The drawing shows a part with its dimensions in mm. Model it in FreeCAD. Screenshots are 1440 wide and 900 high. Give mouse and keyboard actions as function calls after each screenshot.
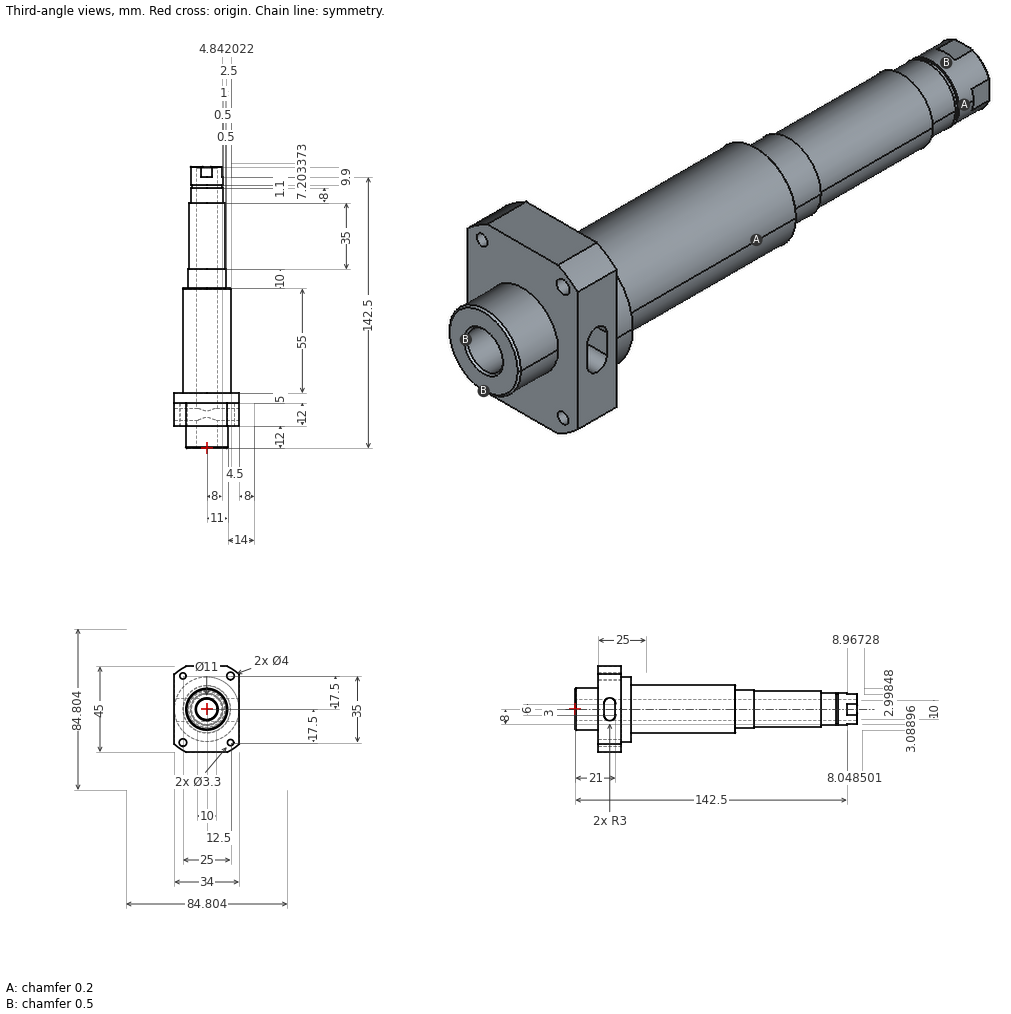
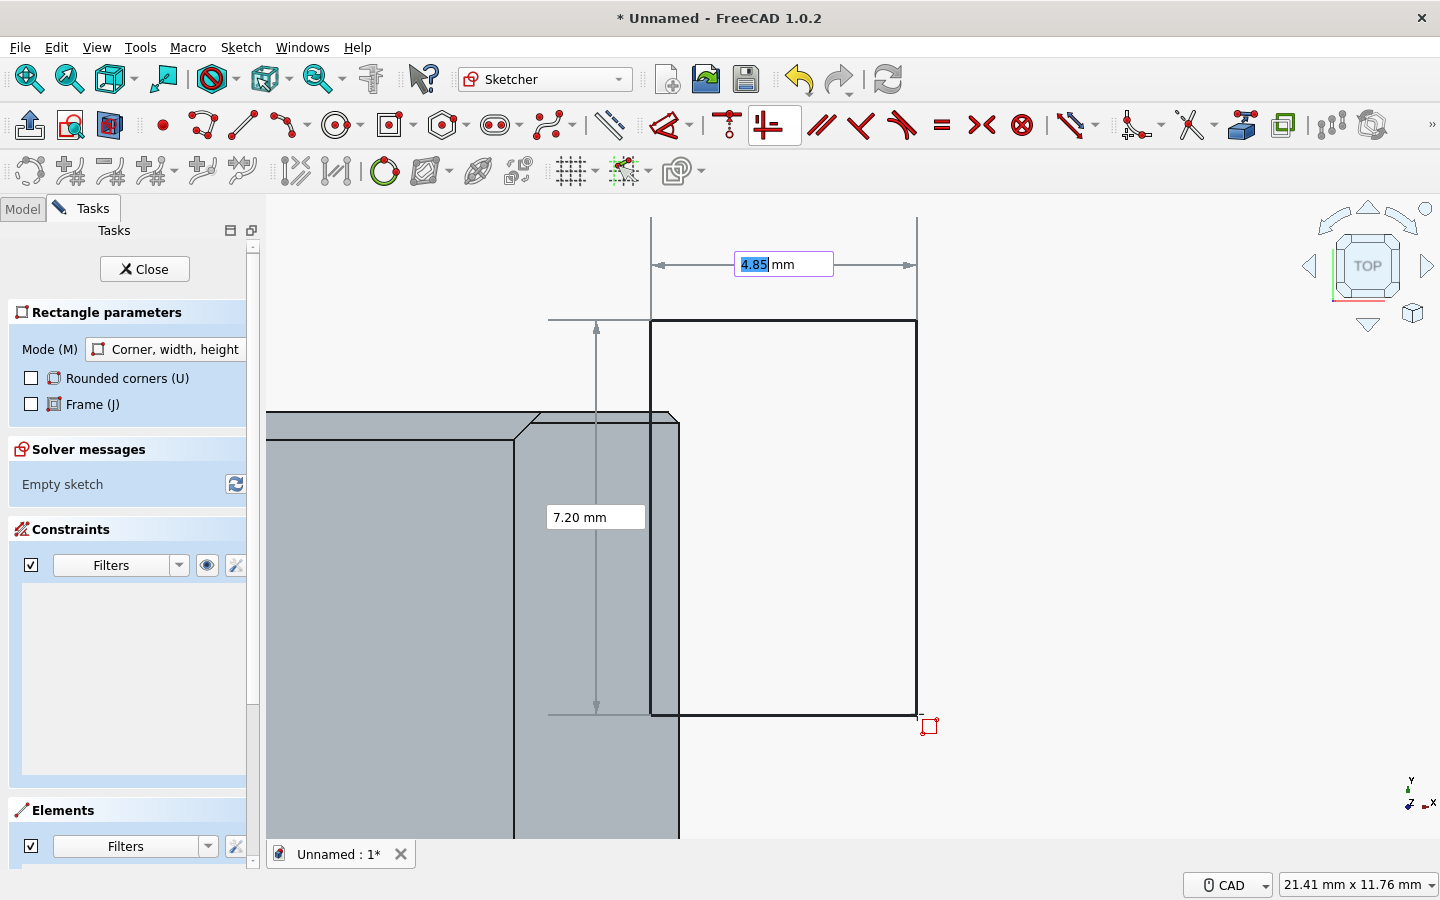
text(4.842022)
key(Tab)
text(7.203373)
key(Return)
key(Escape)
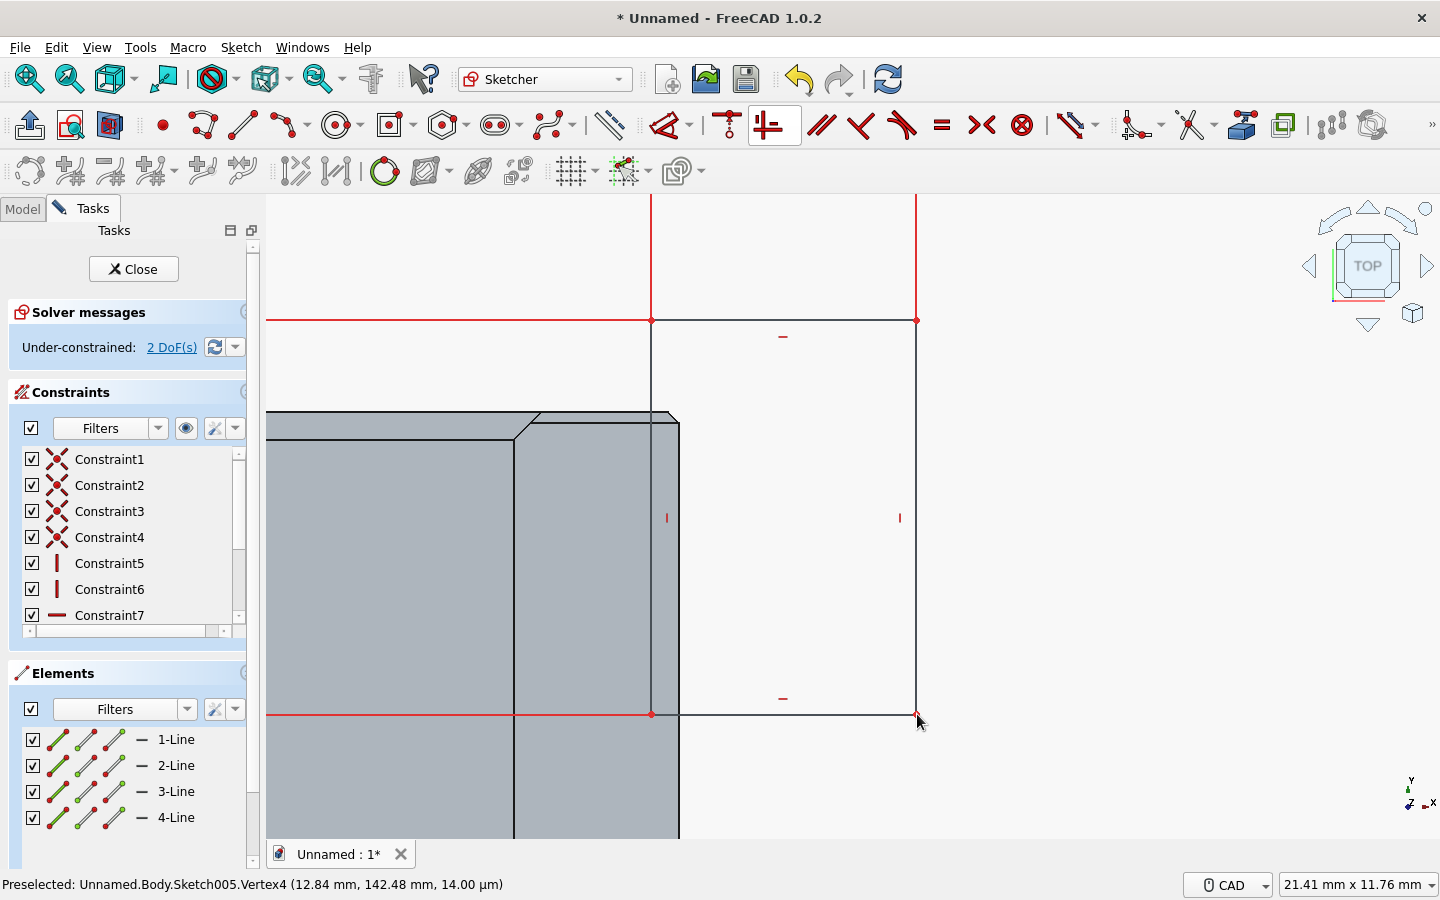
click(664, 126)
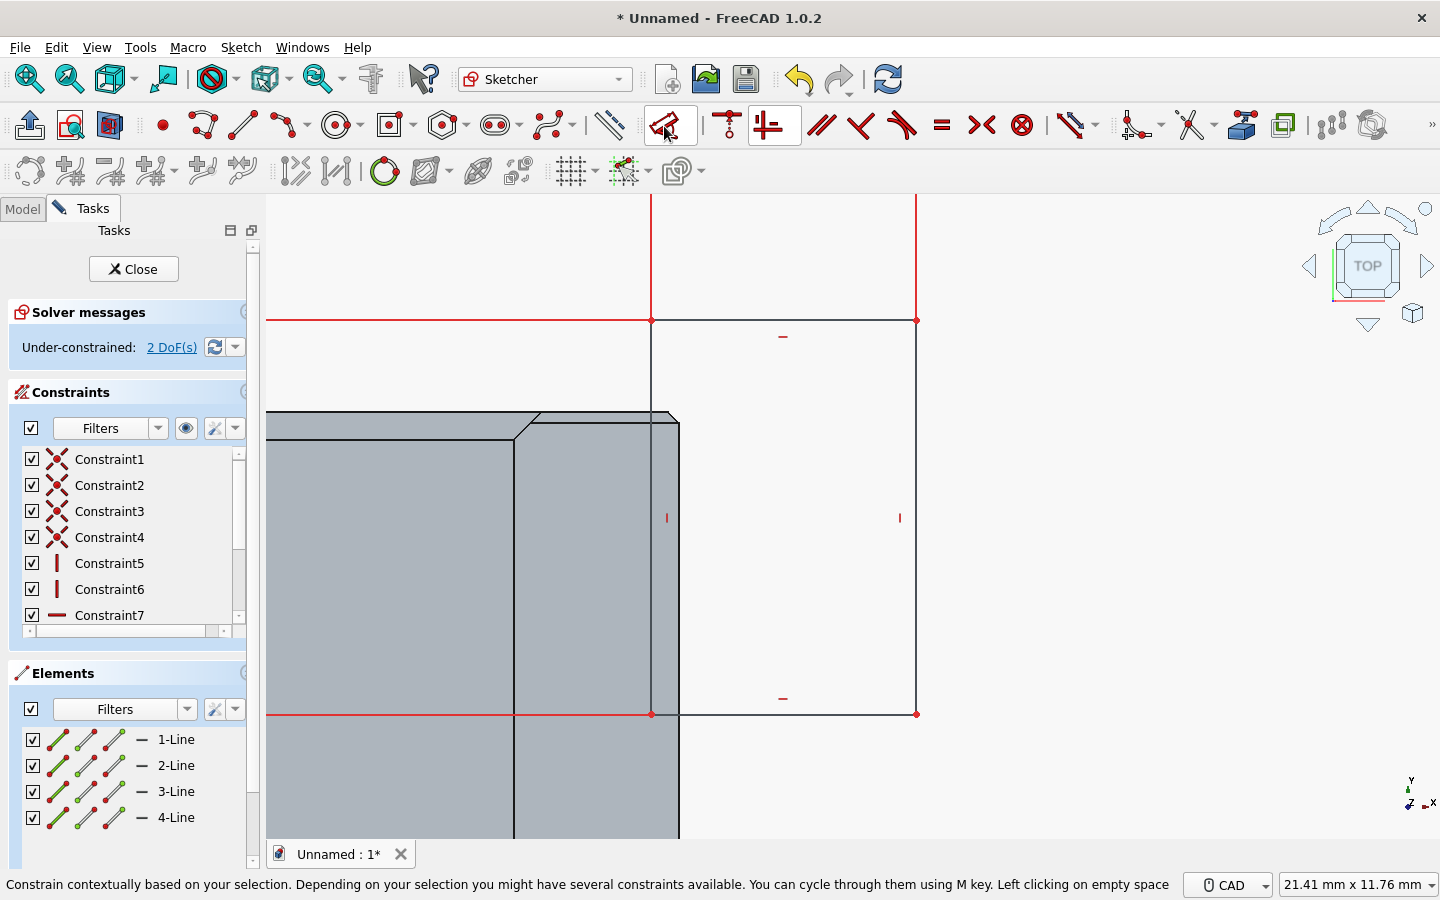
click(651, 320)
click(472, 286)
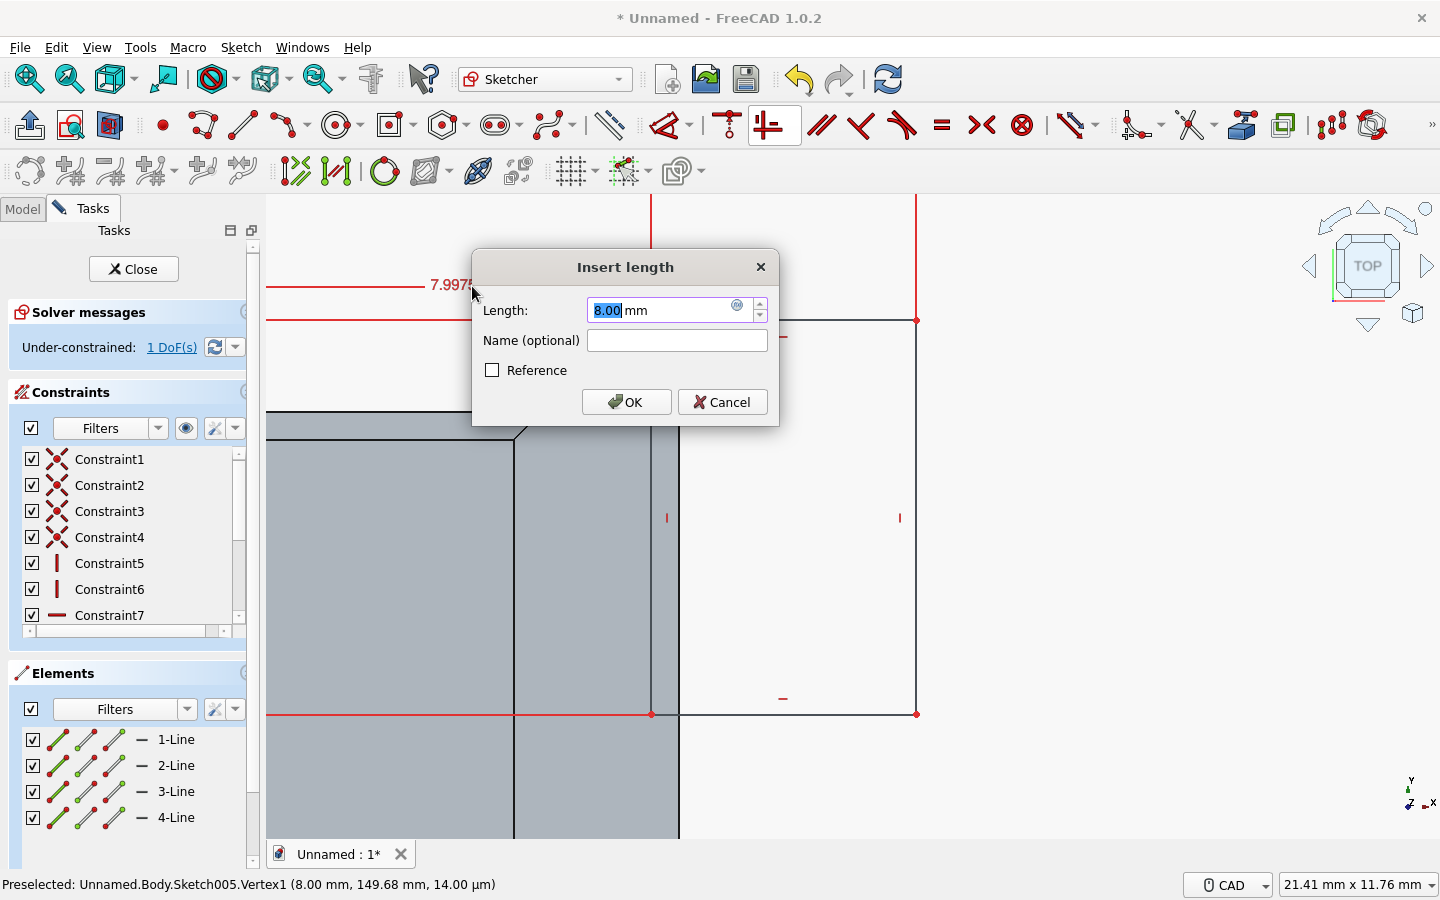
text(8)
key(Return)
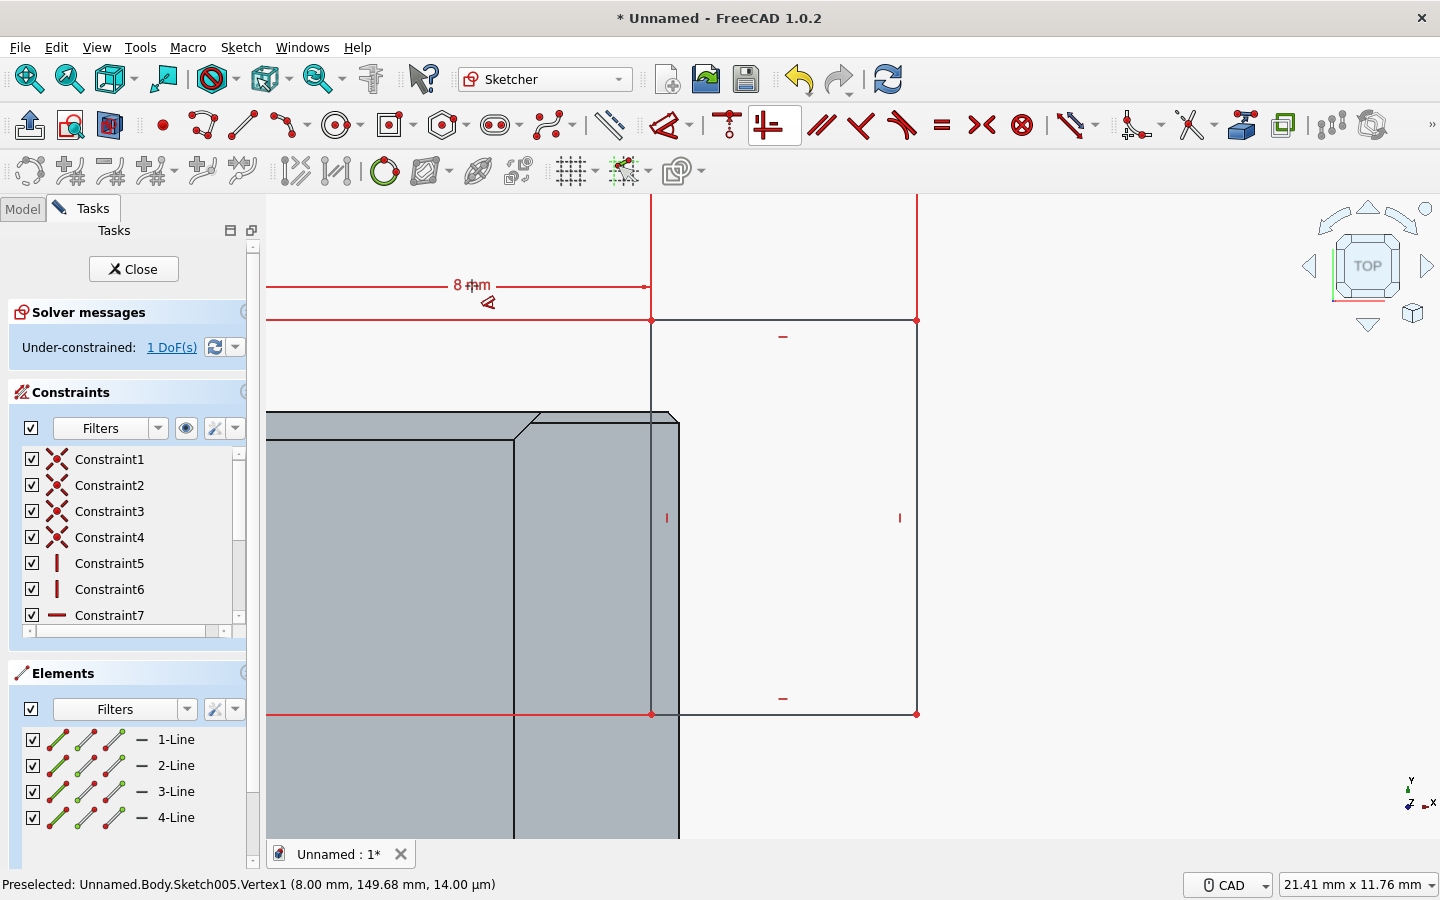
click(651, 715)
click(685, 763)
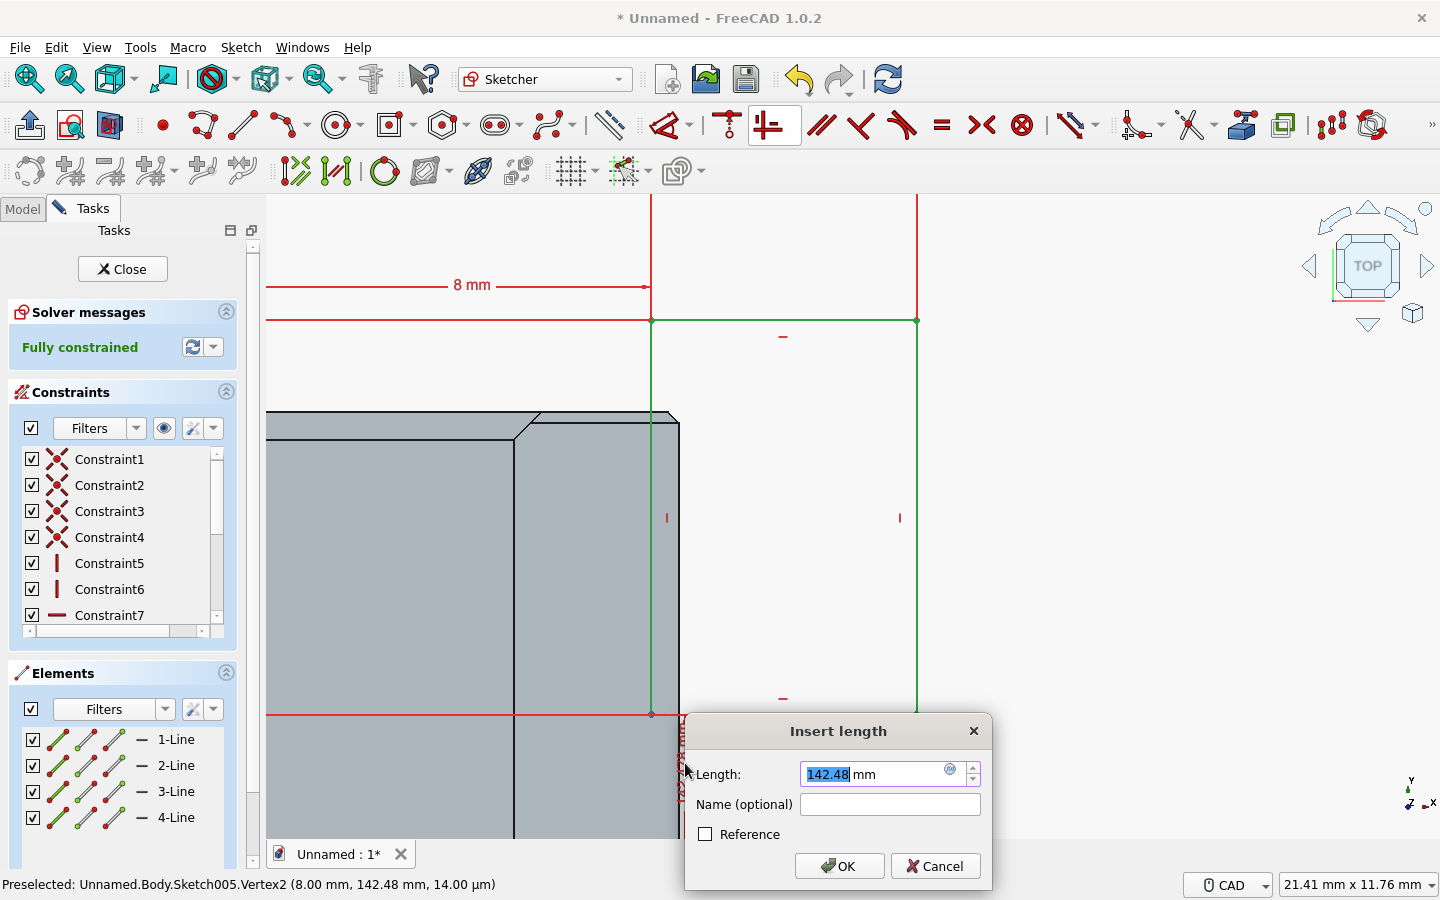
text(142.5)
key(Return)
key(Escape)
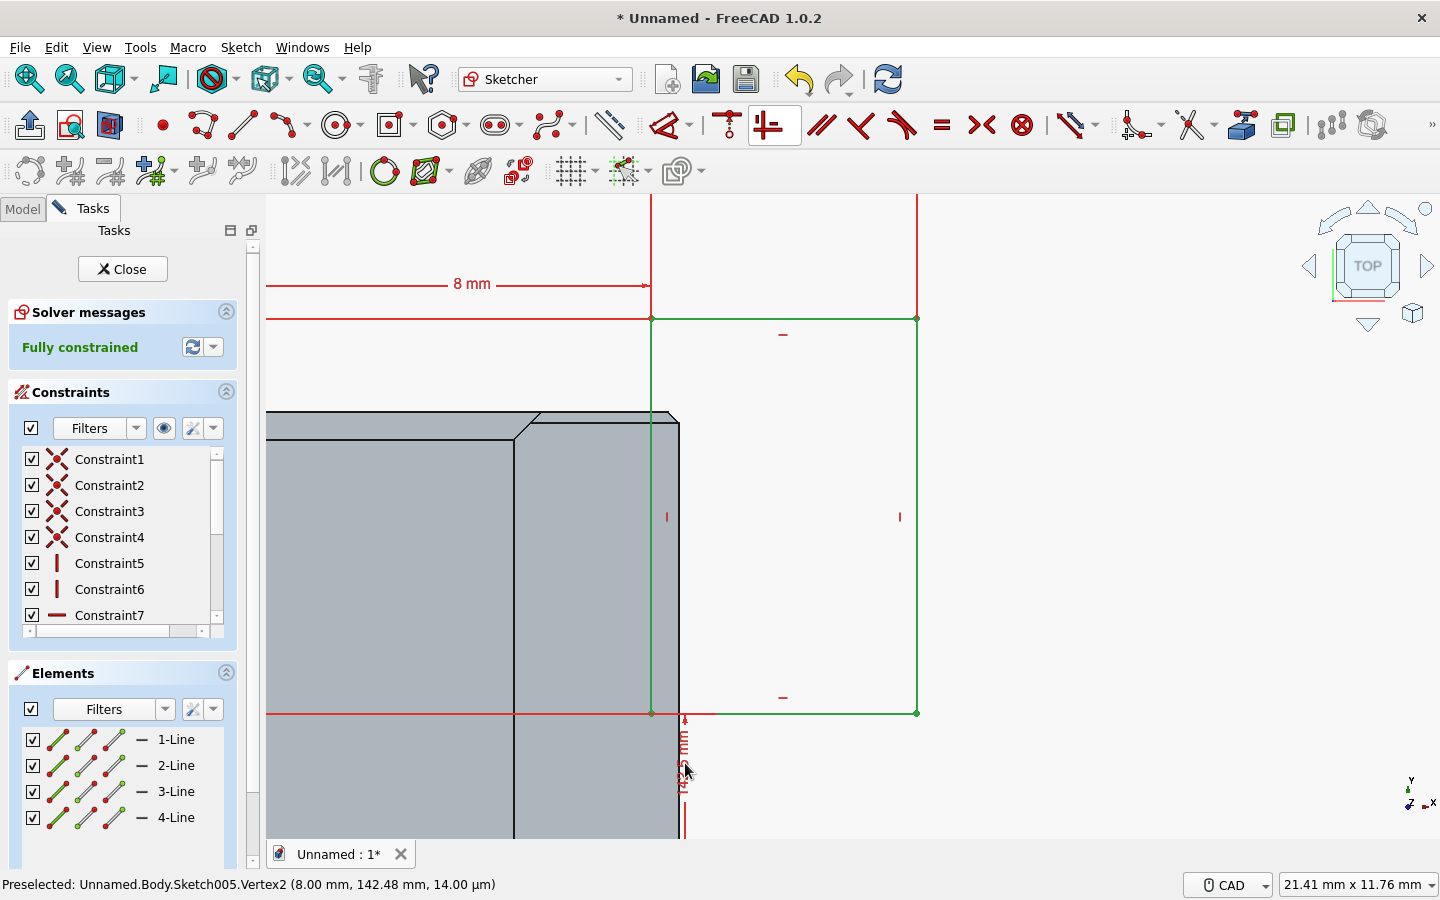
click(123, 269)